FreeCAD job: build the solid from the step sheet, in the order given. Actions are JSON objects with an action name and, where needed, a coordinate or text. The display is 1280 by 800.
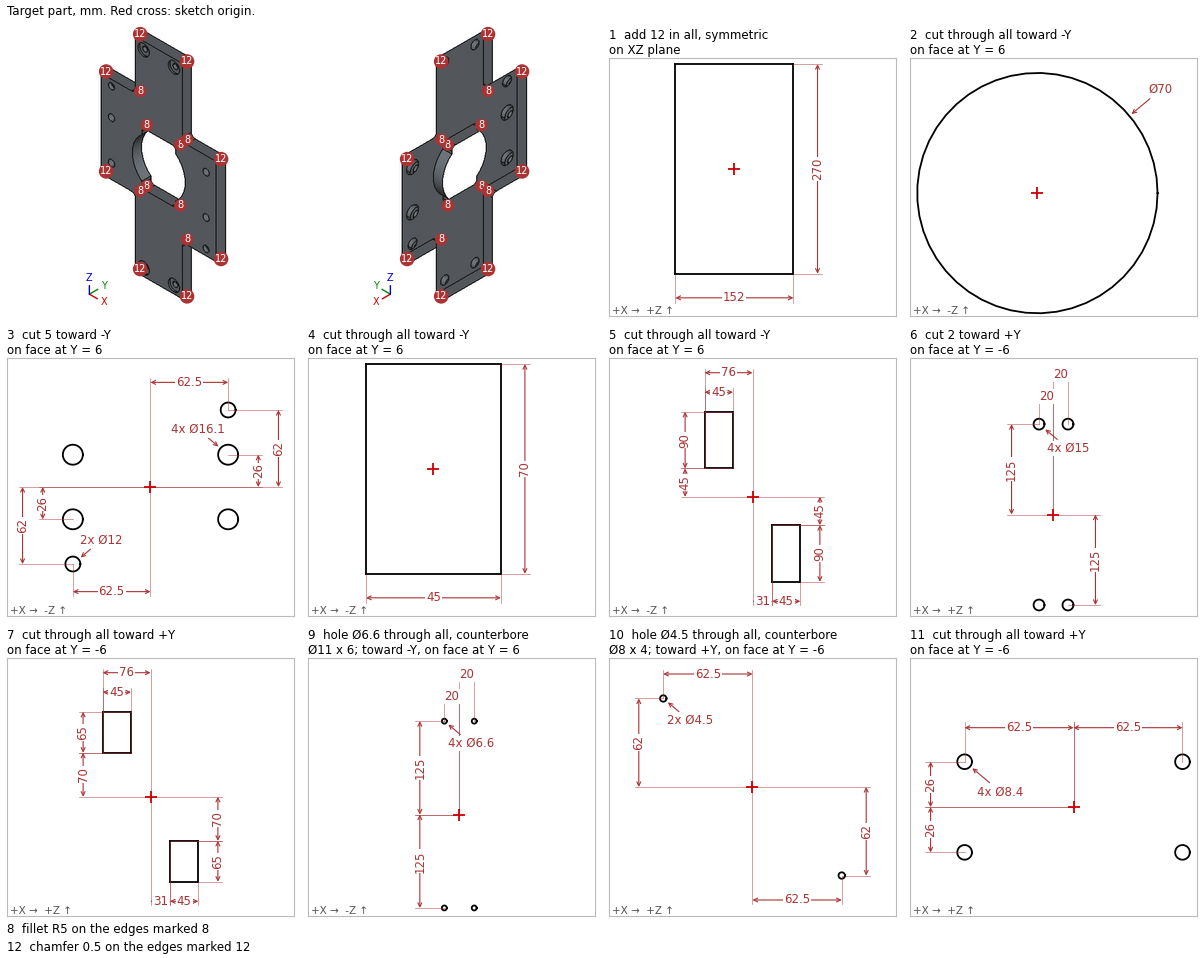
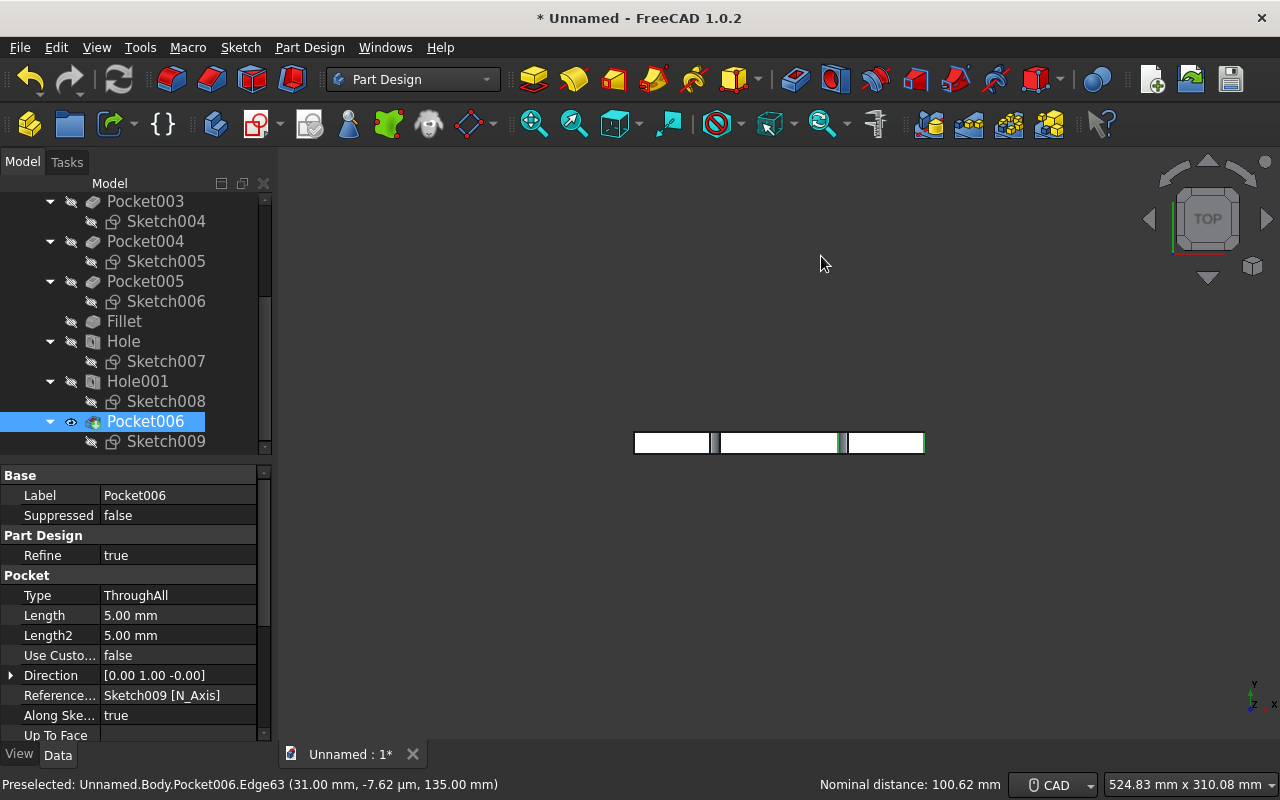
{"action": "key", "text": "v f"}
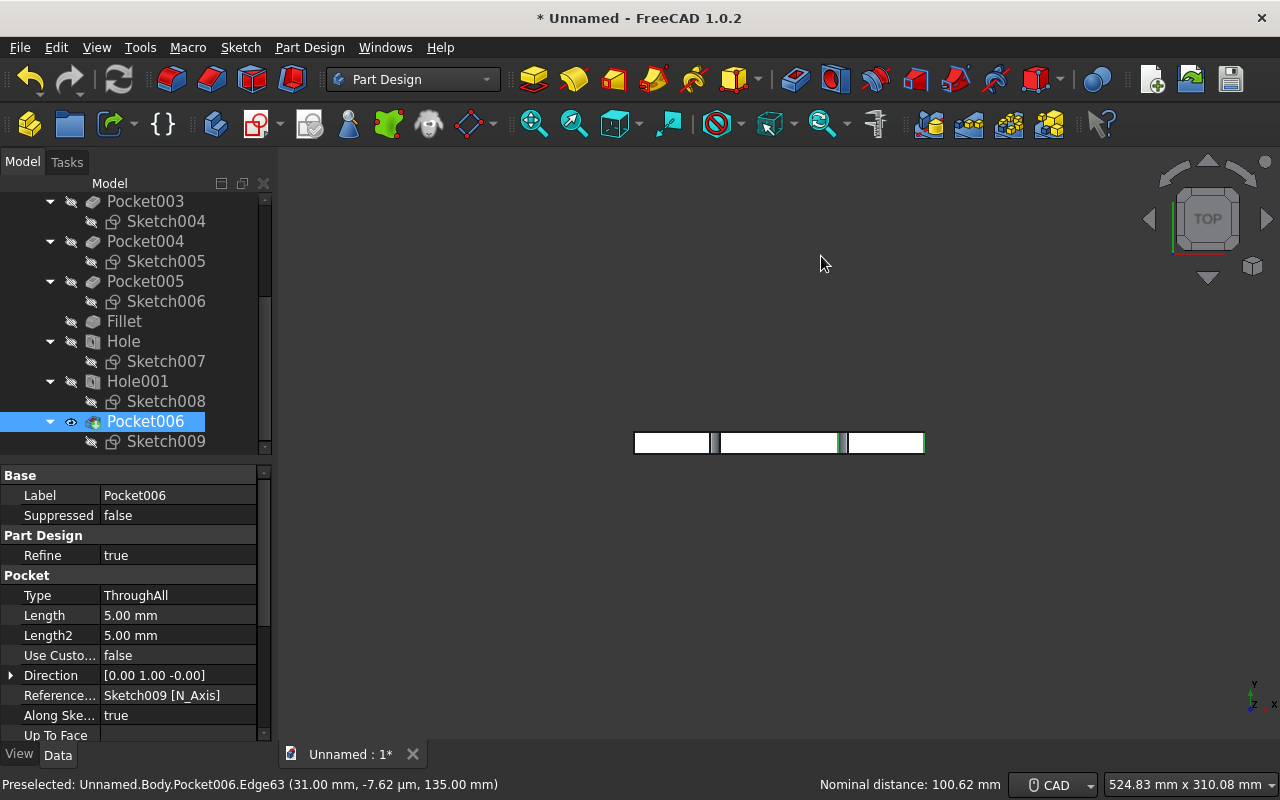
{"action": "left_click", "coordinate": [634, 442], "text": "ctrl"}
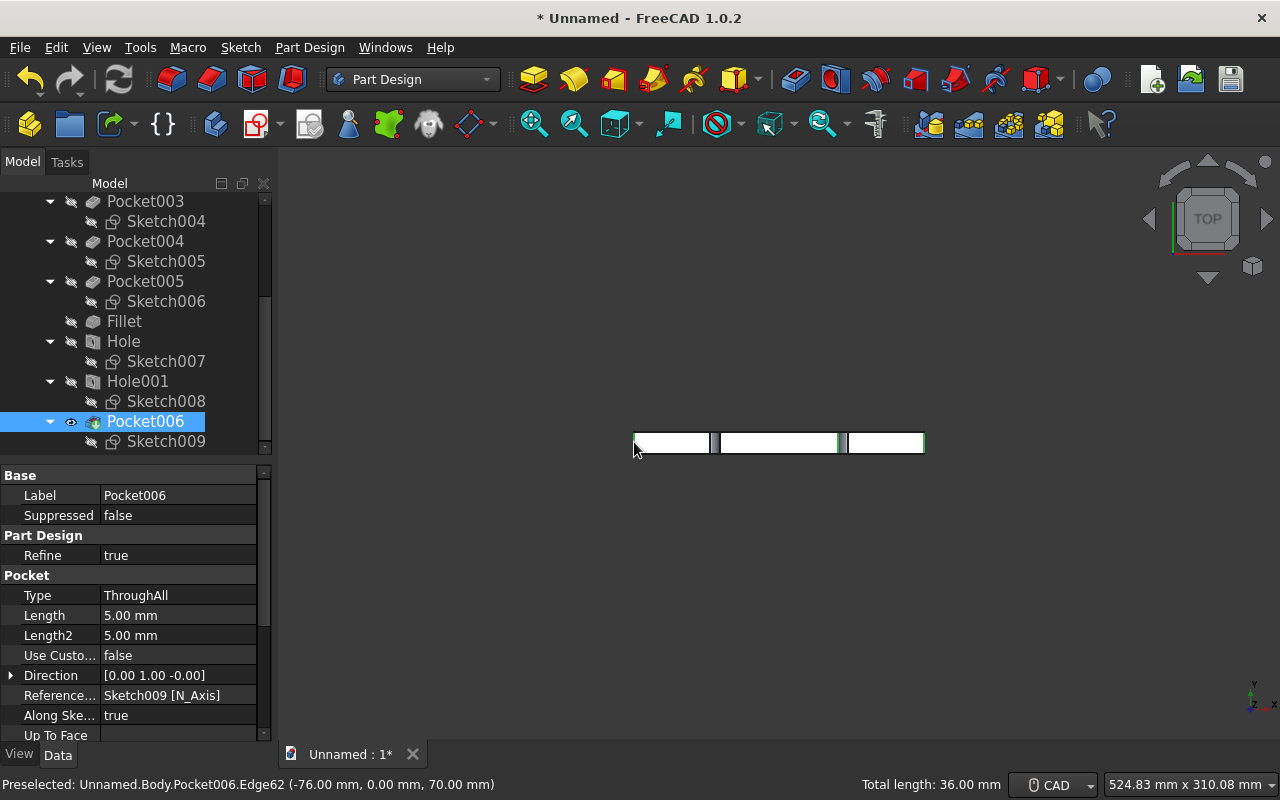
{"action": "left_click", "coordinate": [720, 442], "text": "ctrl"}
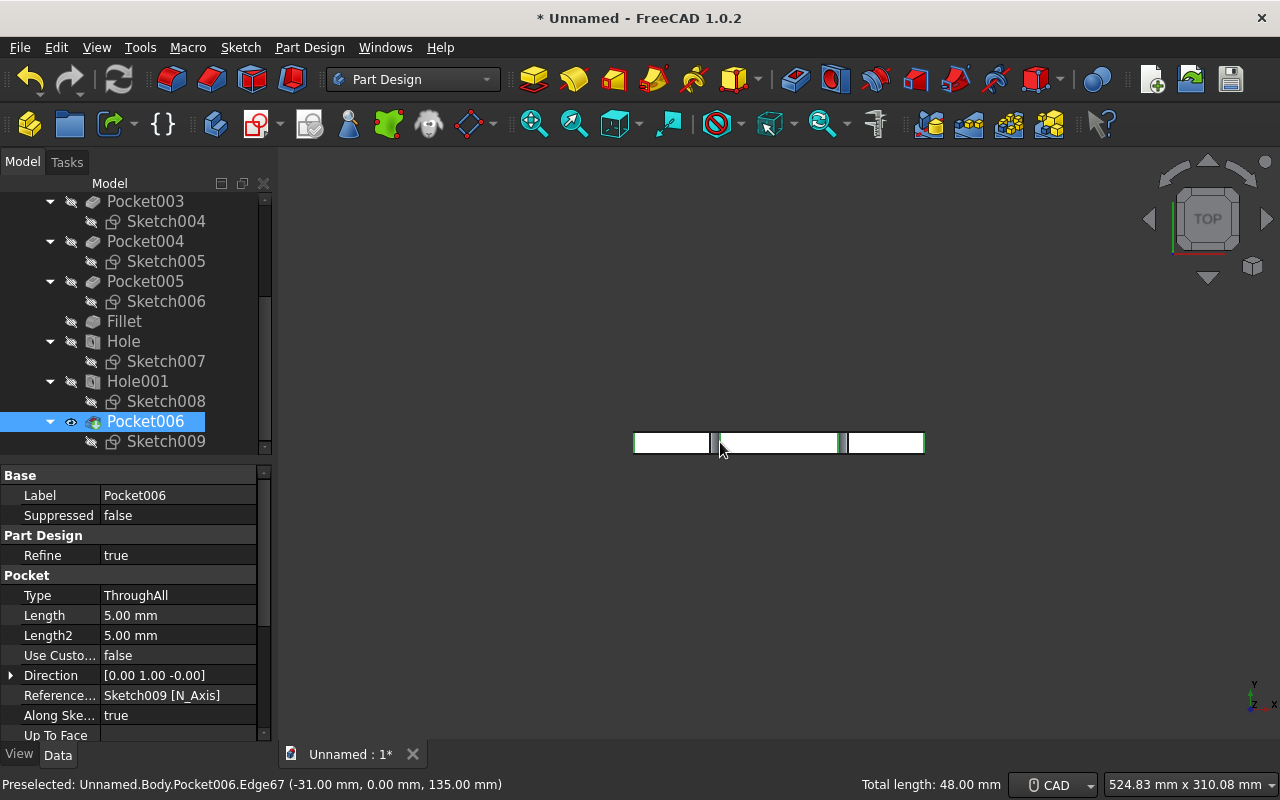
{"action": "key", "text": "0"}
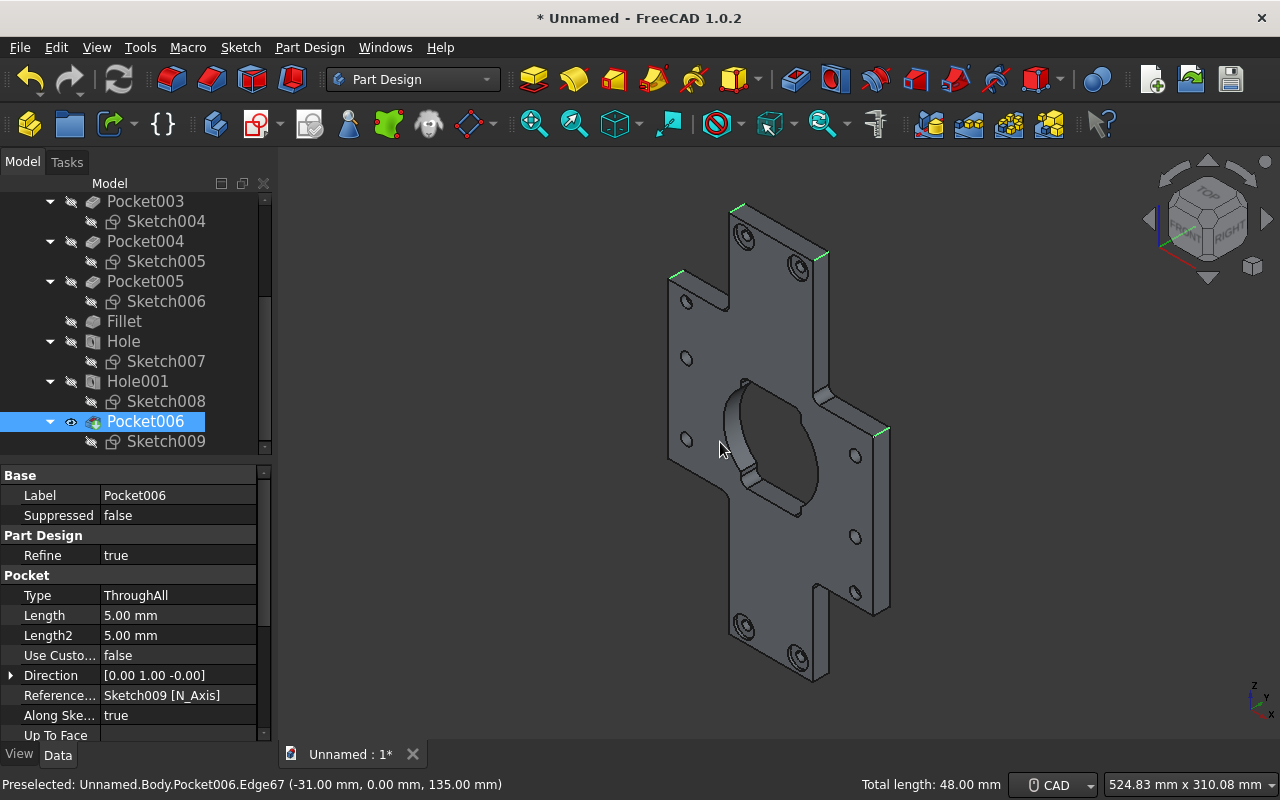
{"action": "key", "text": "1"}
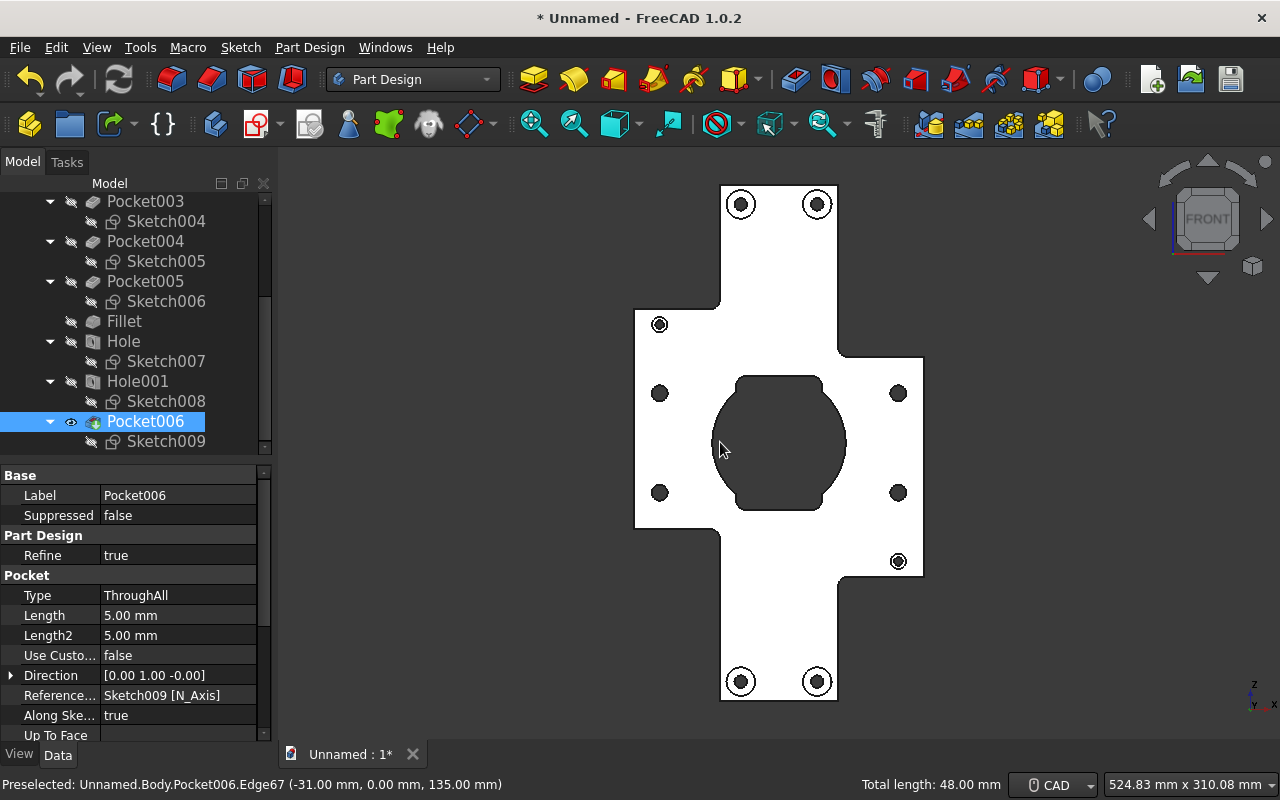
{"action": "key", "text": "3"}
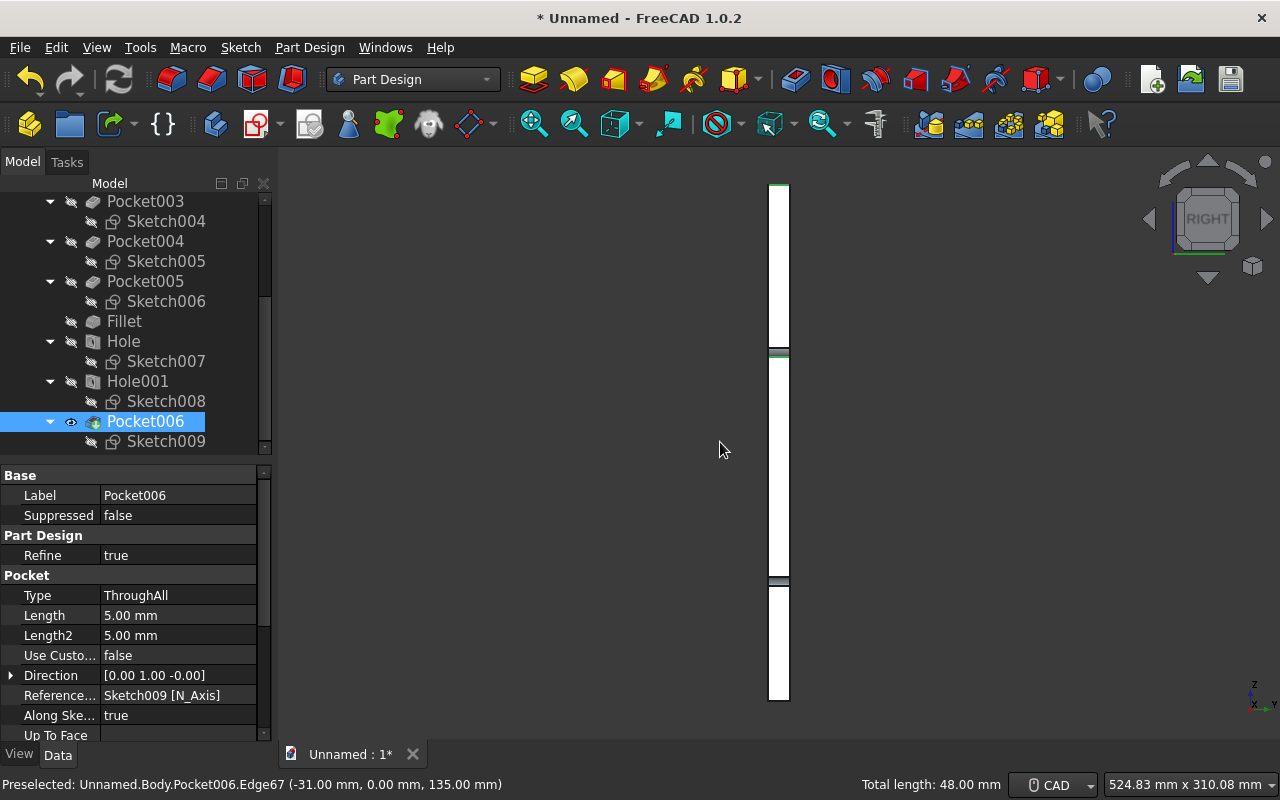
{"action": "left_click", "coordinate": [779, 576], "text": "ctrl"}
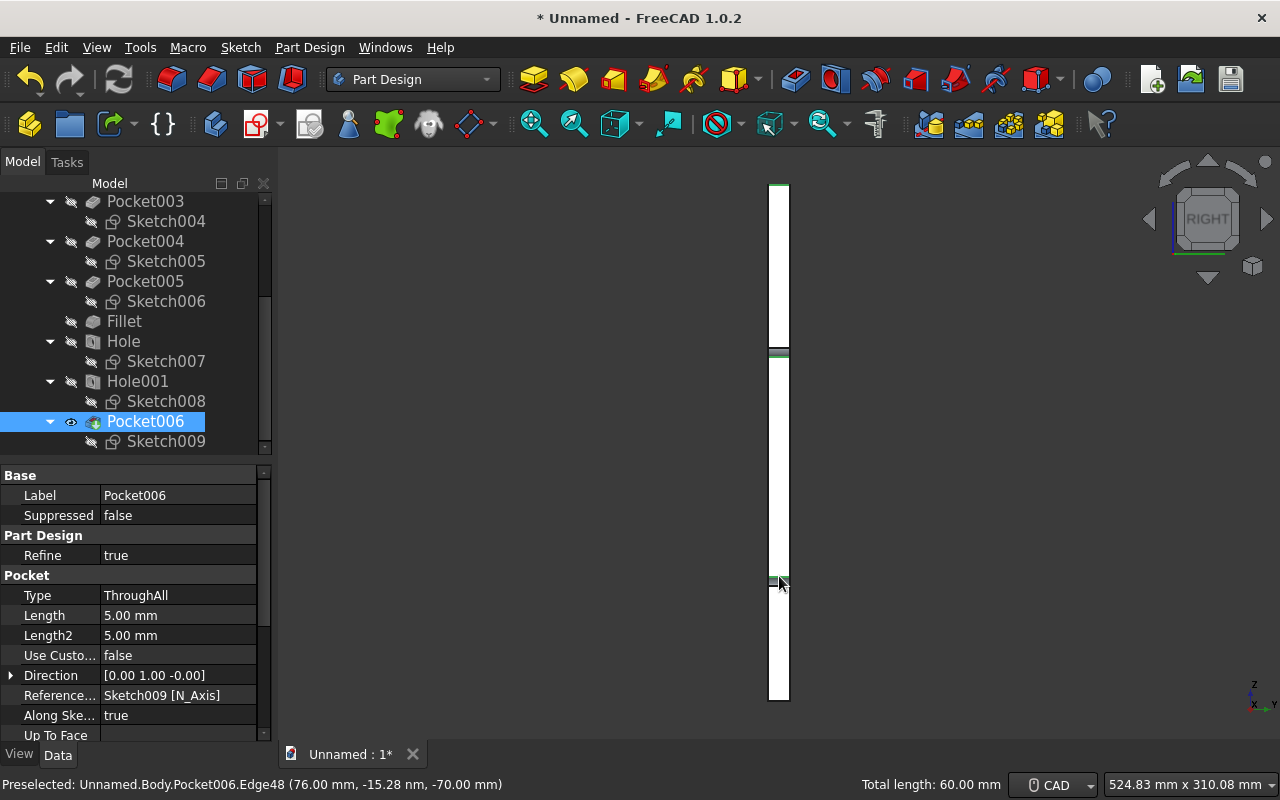
{"action": "left_click", "coordinate": [779, 700], "text": "ctrl"}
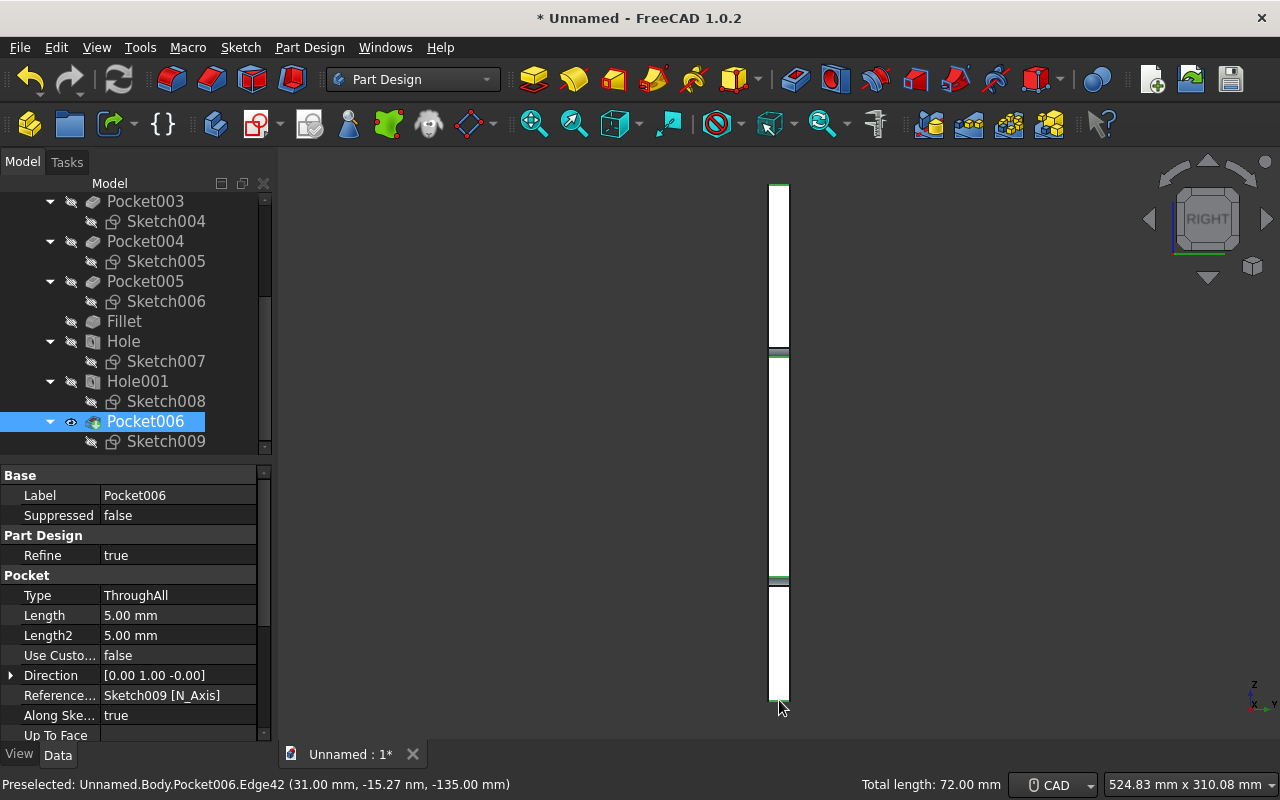
{"action": "key", "text": "5"}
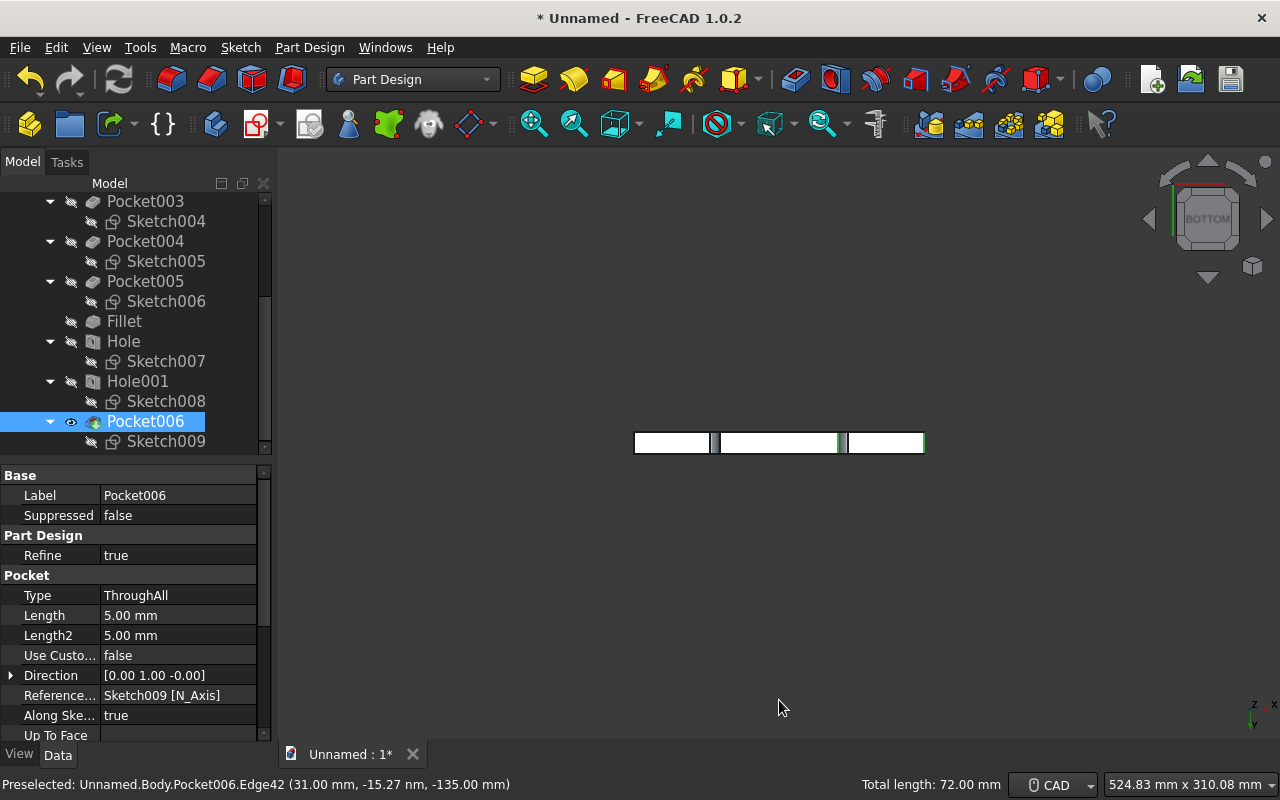
{"action": "key", "text": "v f"}